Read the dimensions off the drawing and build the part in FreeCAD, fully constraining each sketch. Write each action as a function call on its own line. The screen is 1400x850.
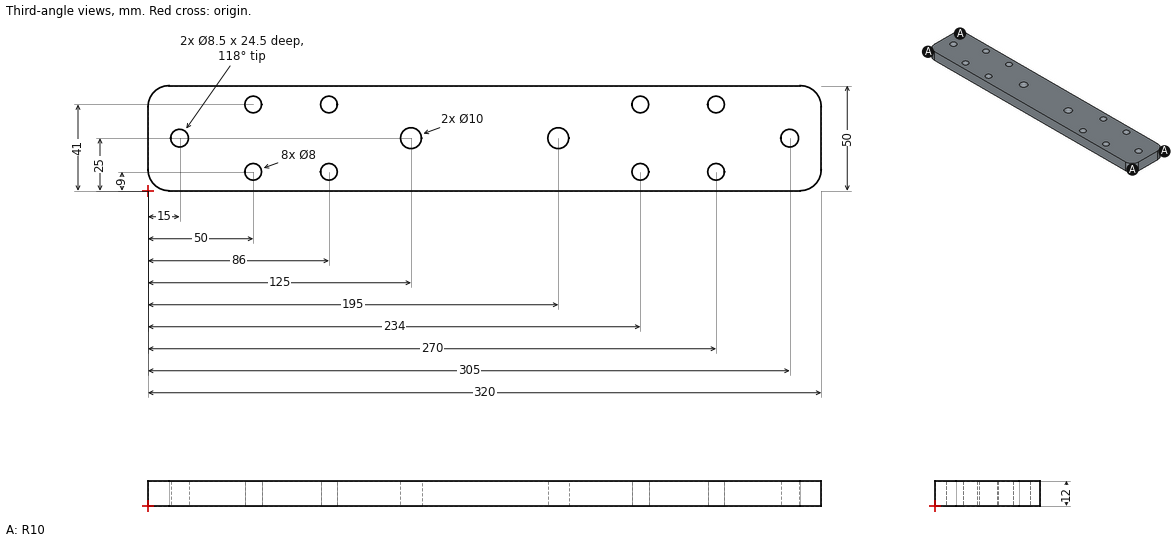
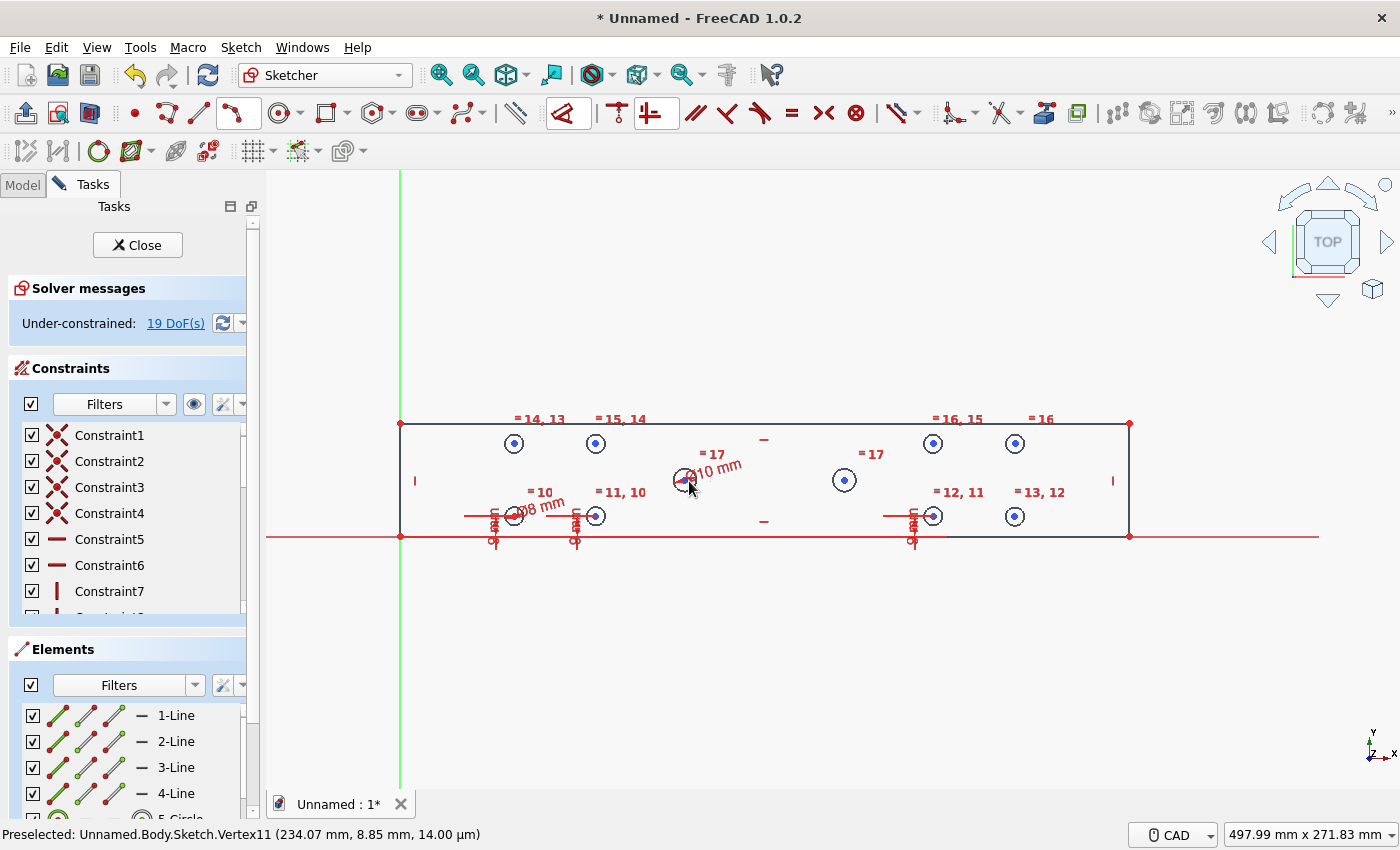
scroll(1015, 517, up, 4)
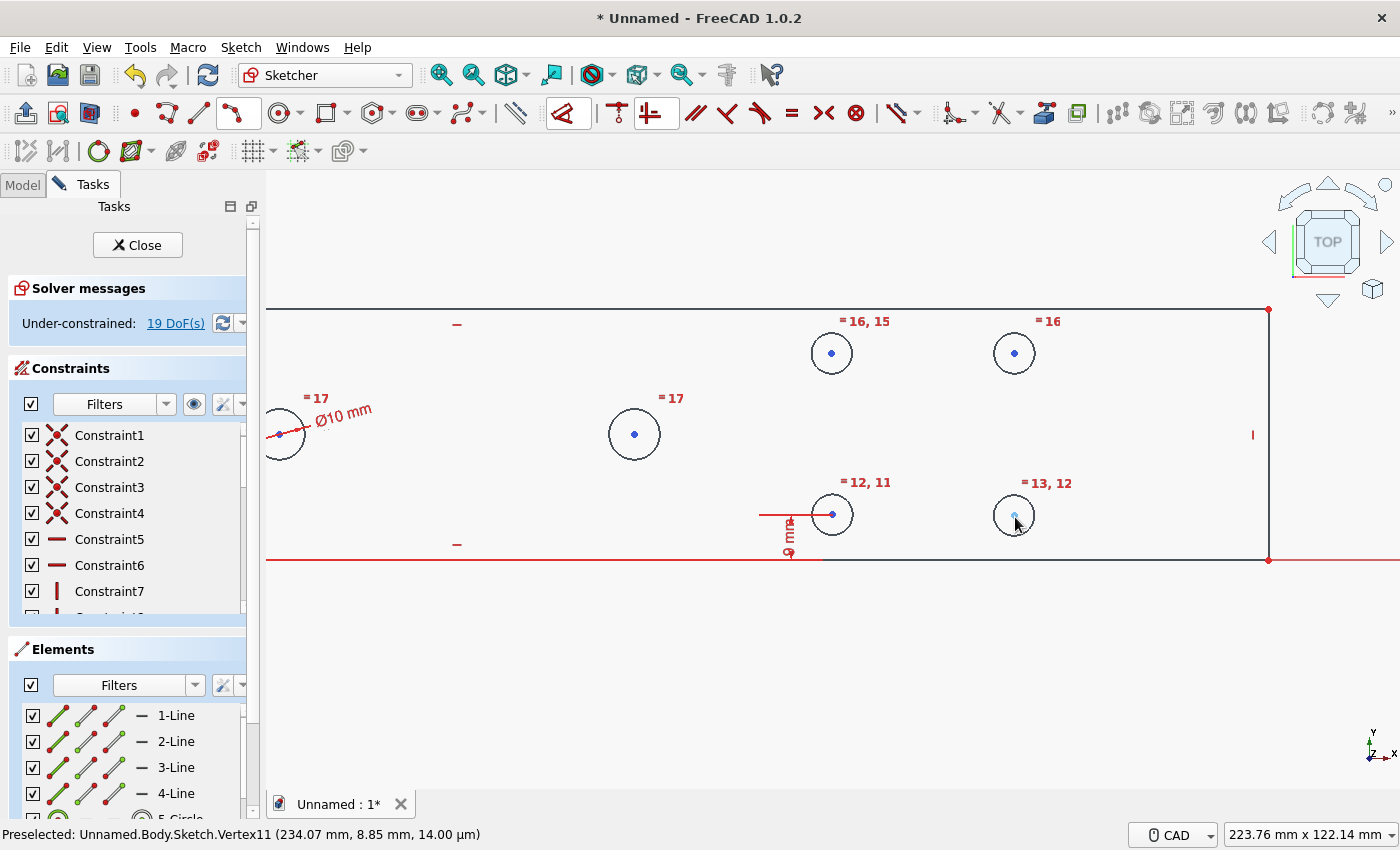
click(1014, 515)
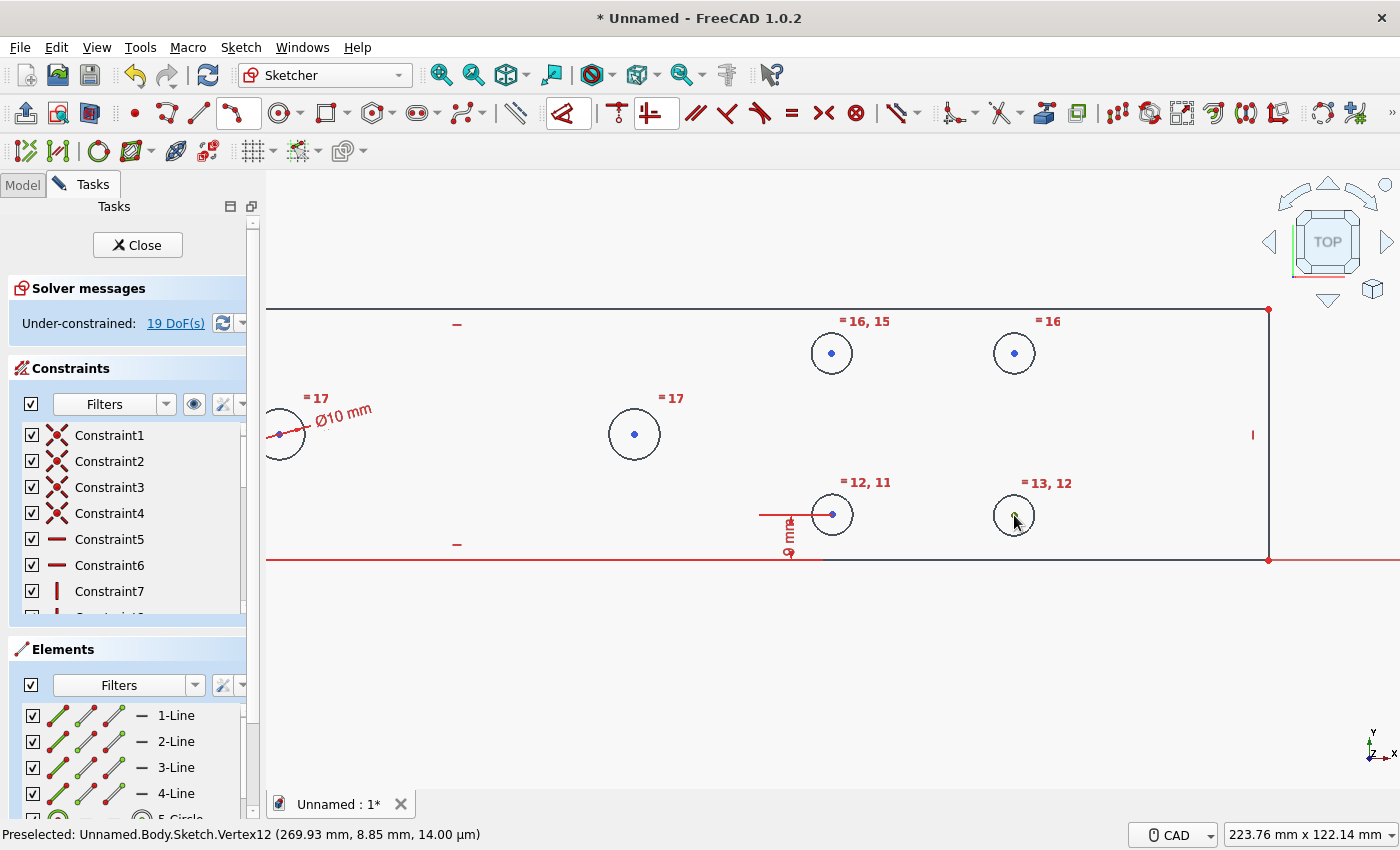
key(i)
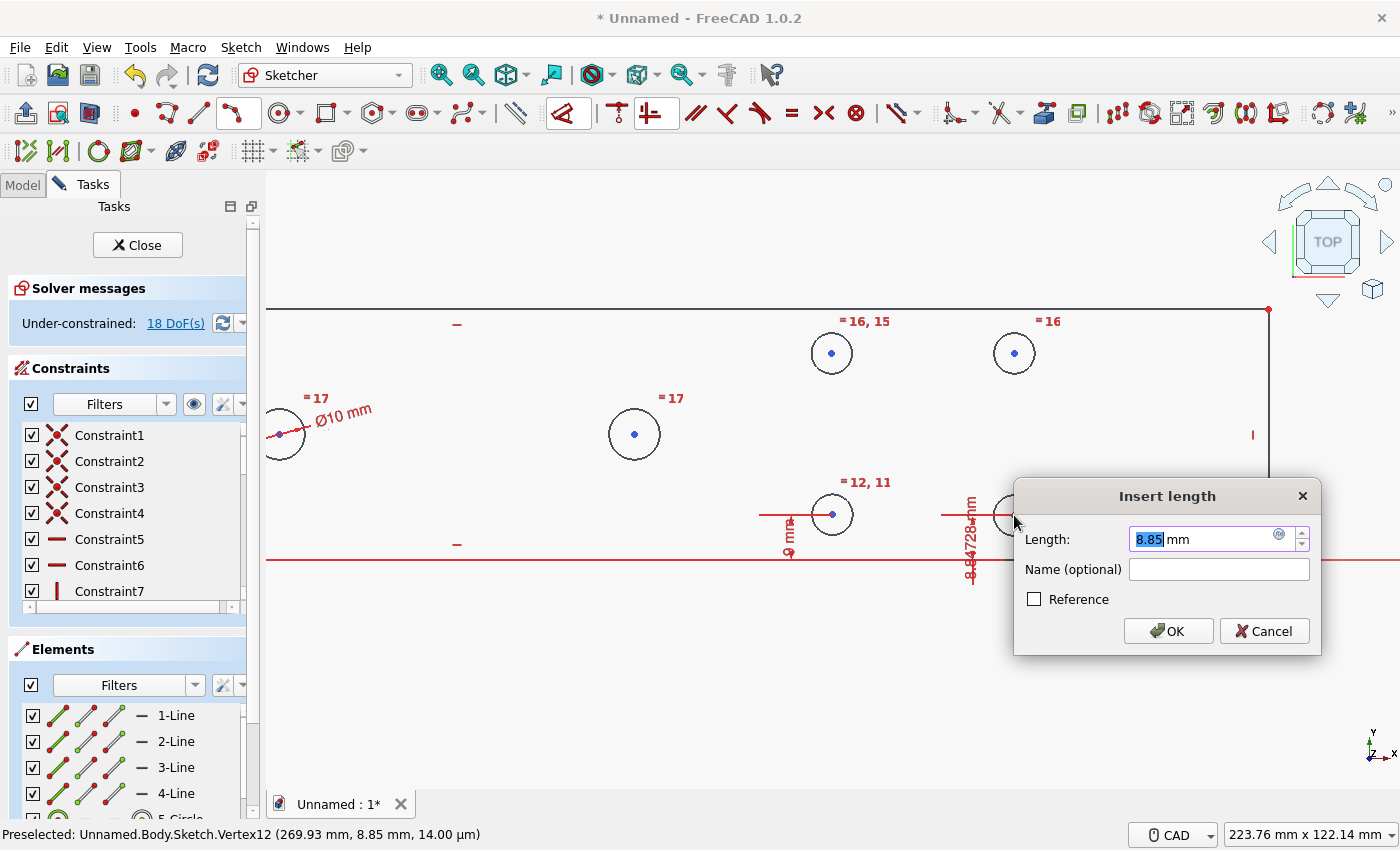
text(9)
key(Return)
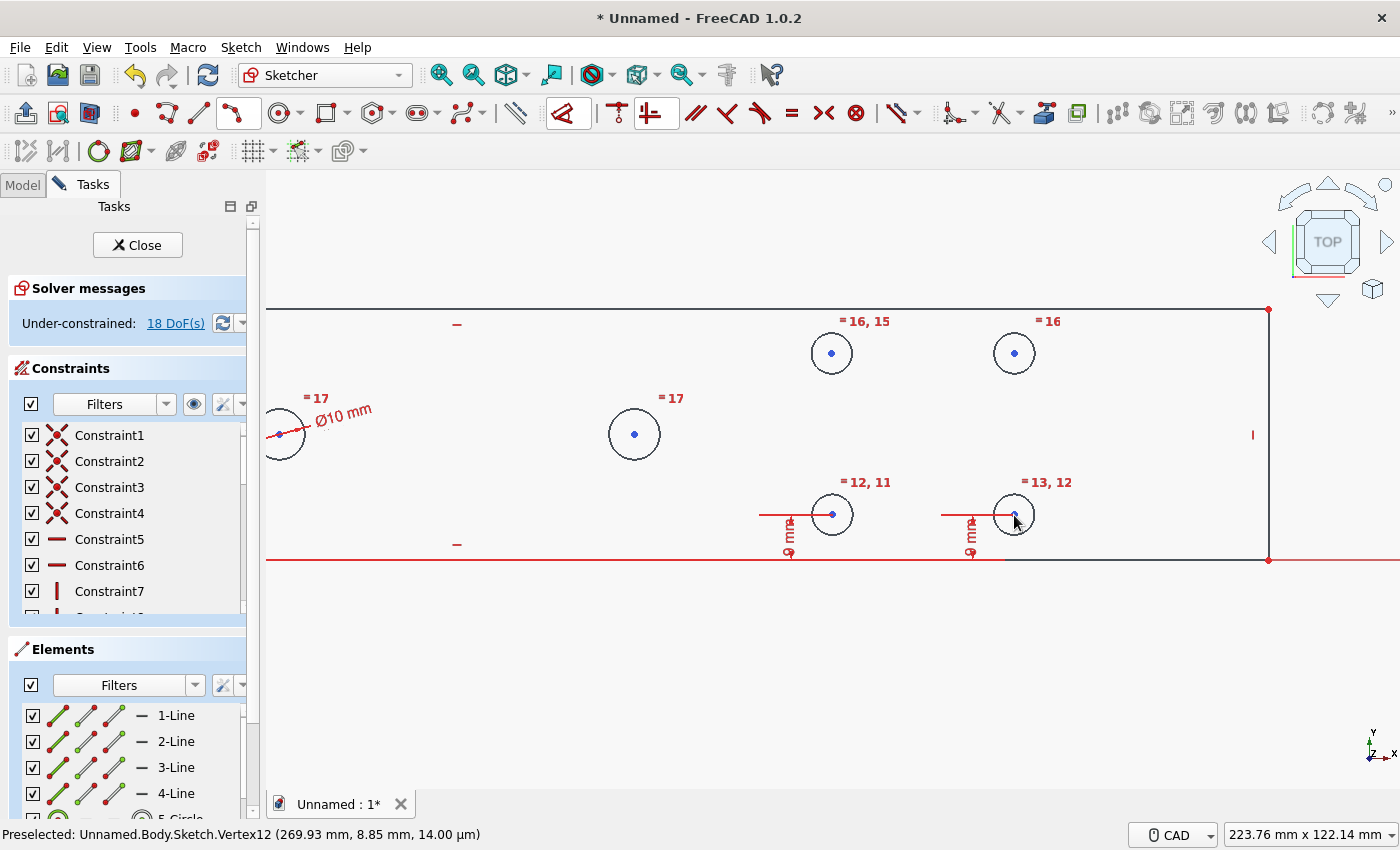
scroll(1015, 517, down, 4)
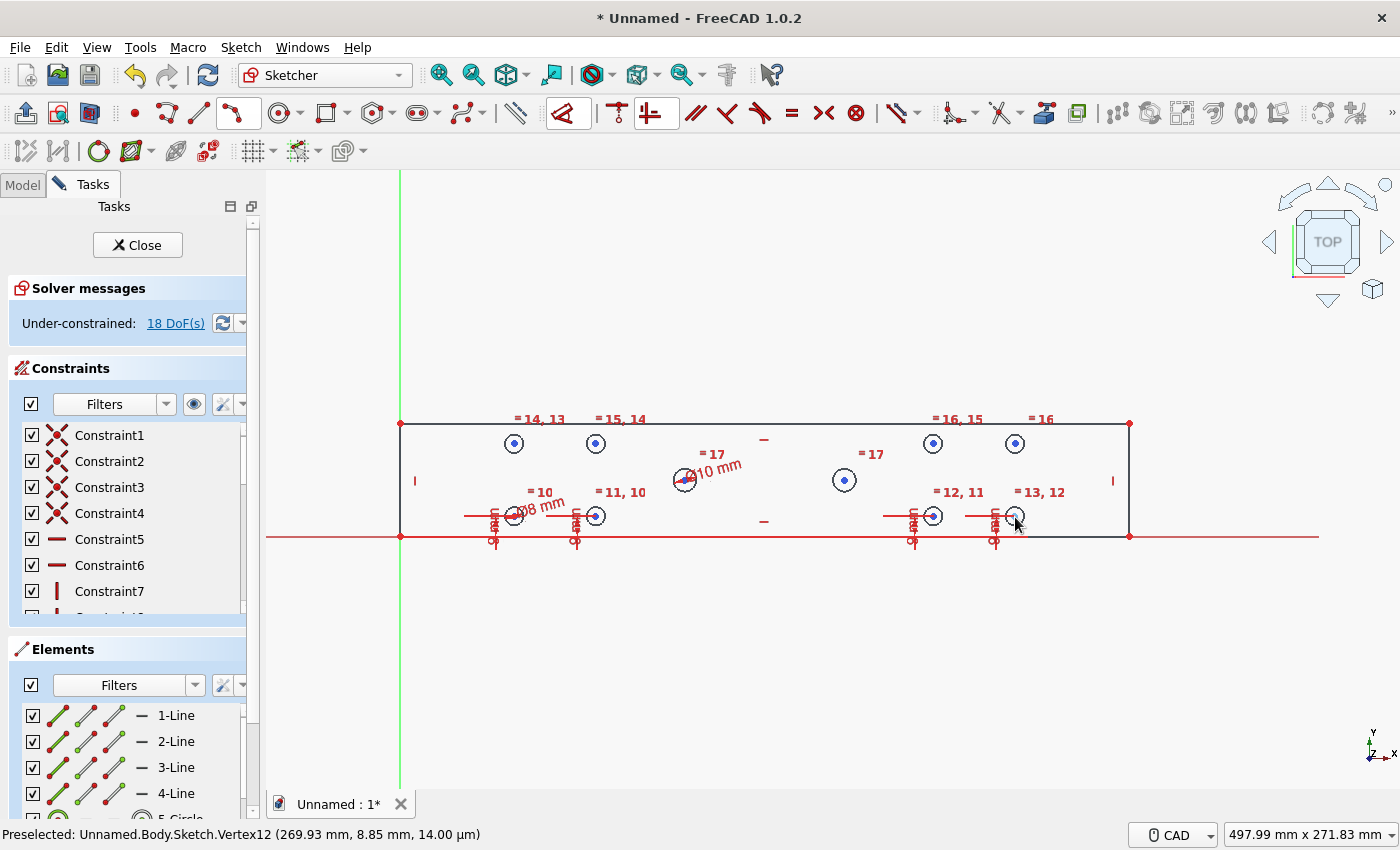
click(1129, 503)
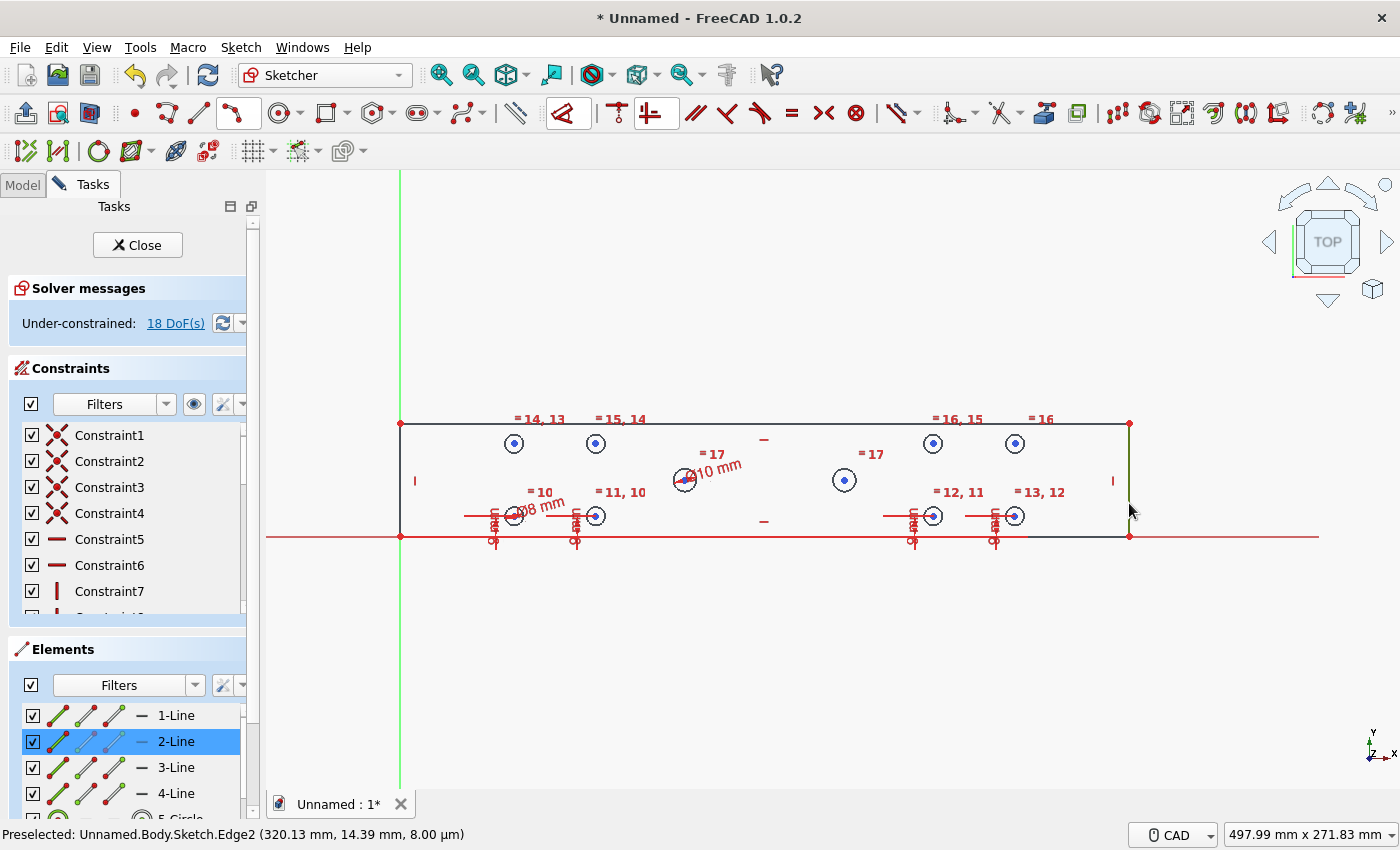
click(586, 114)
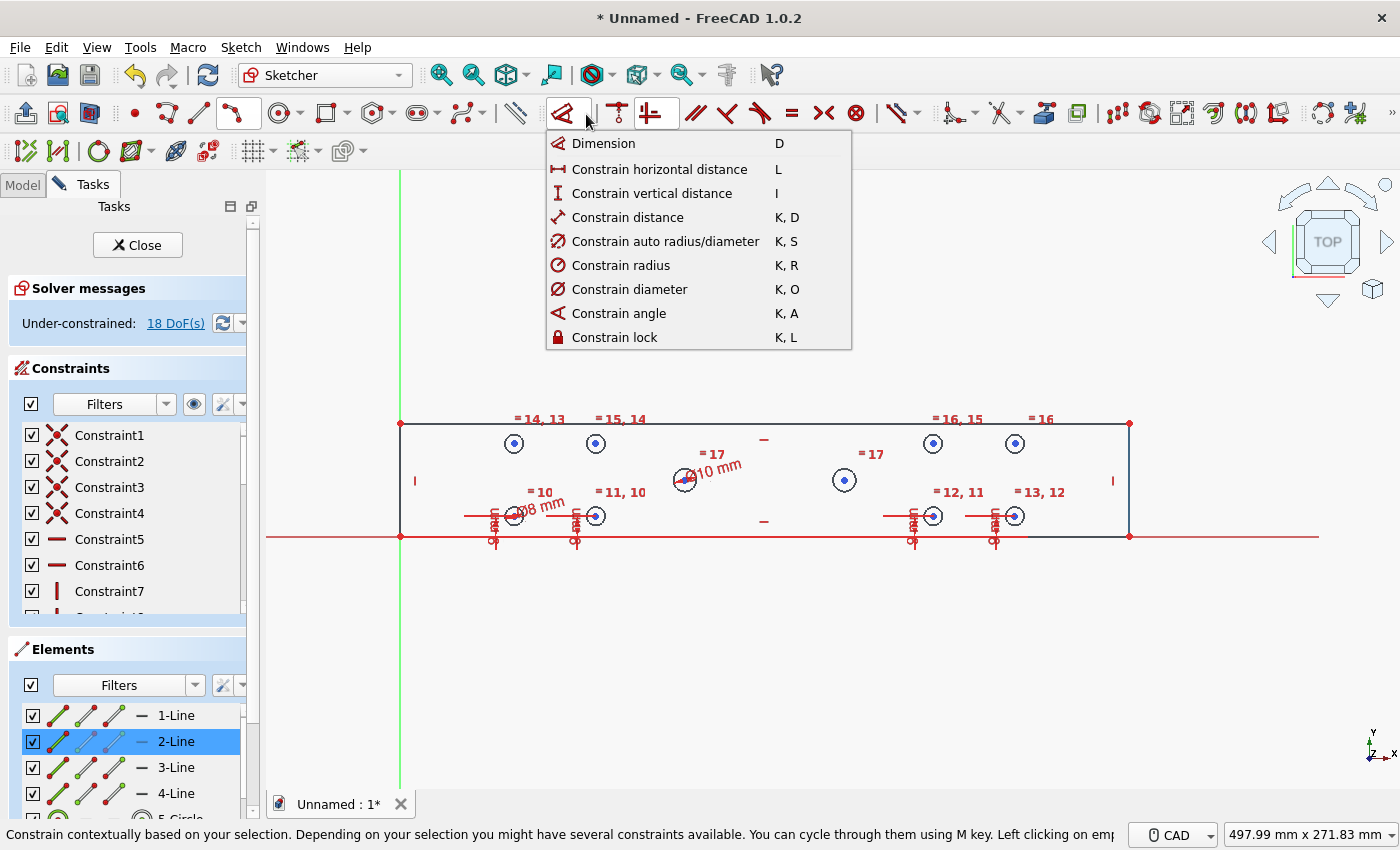
click(699, 193)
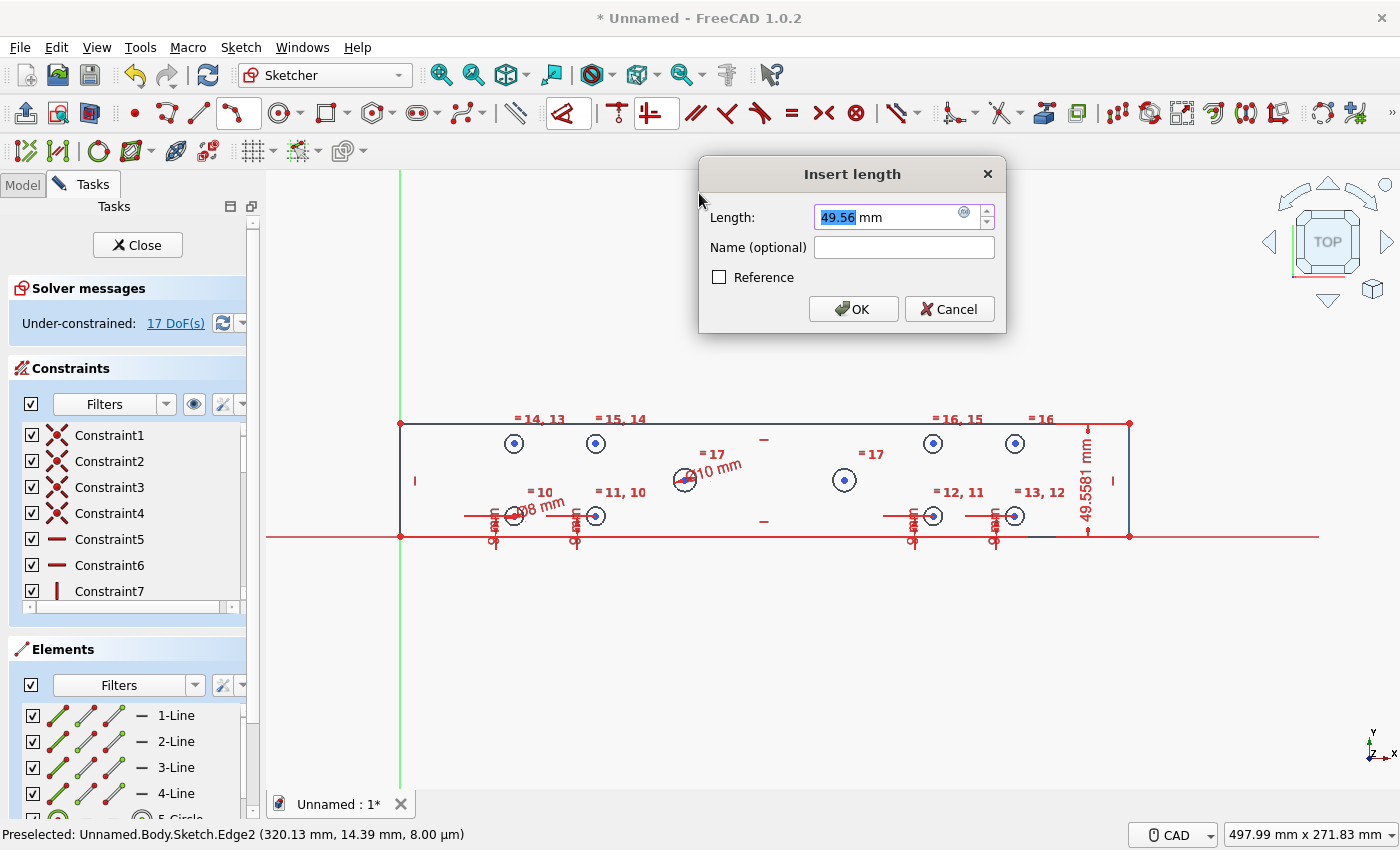
text(50)
key(Return)